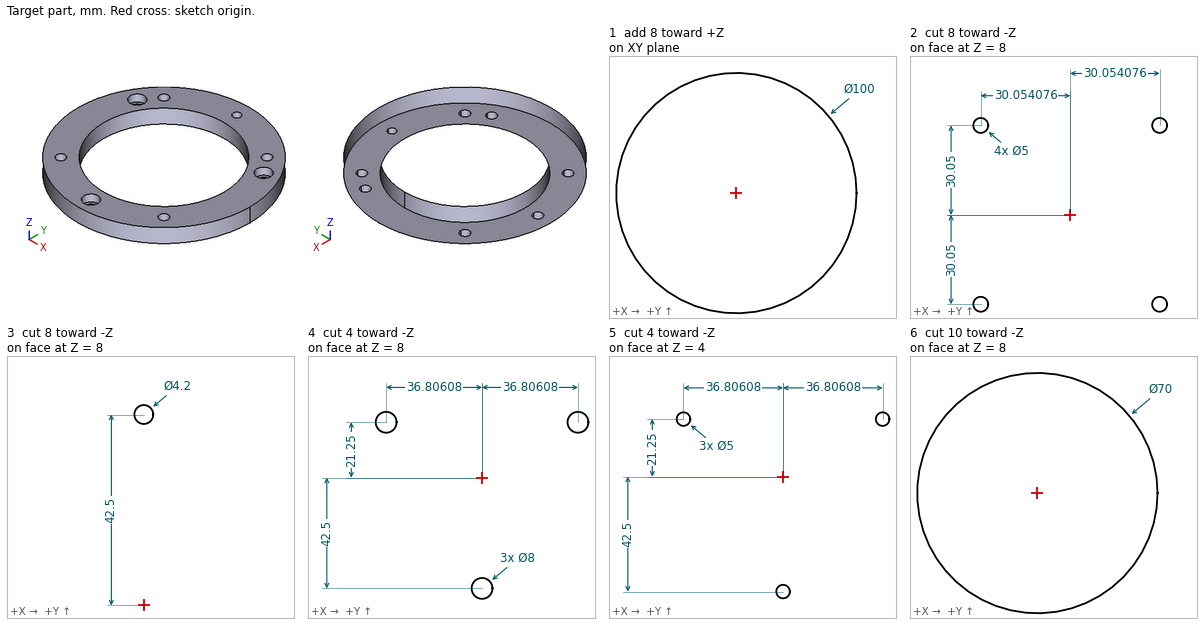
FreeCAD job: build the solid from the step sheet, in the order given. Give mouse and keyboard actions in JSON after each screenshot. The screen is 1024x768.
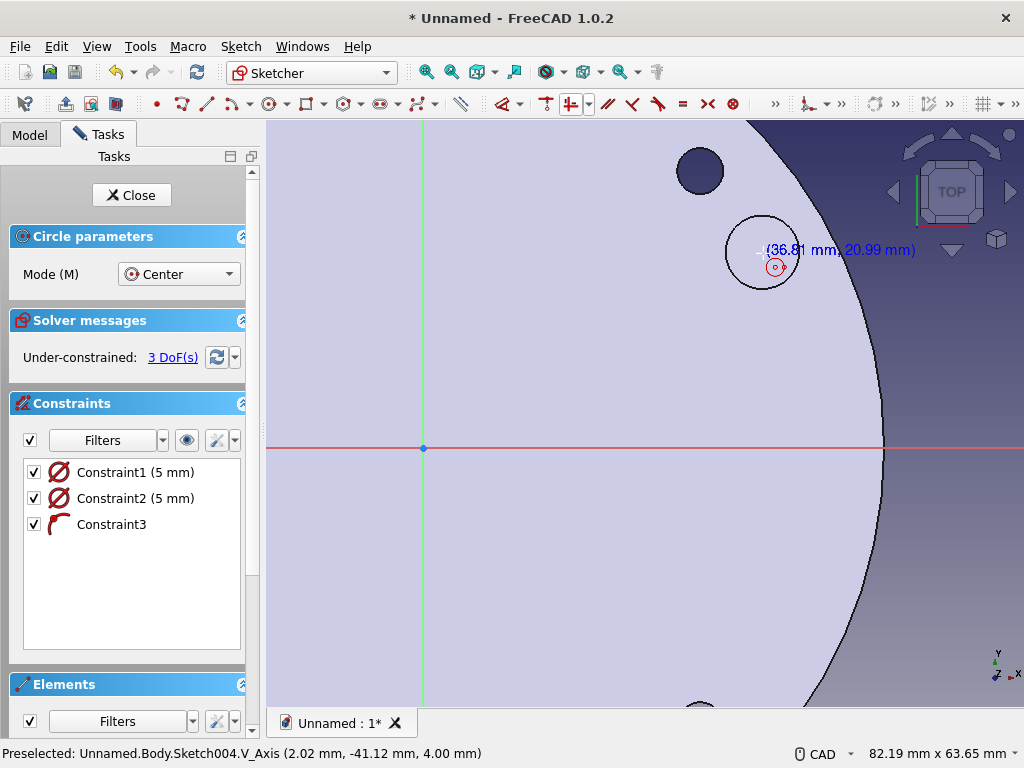
{"action": "left_click", "coordinate": [762, 252]}
{"action": "mouse_move", "coordinate": [779, 236]}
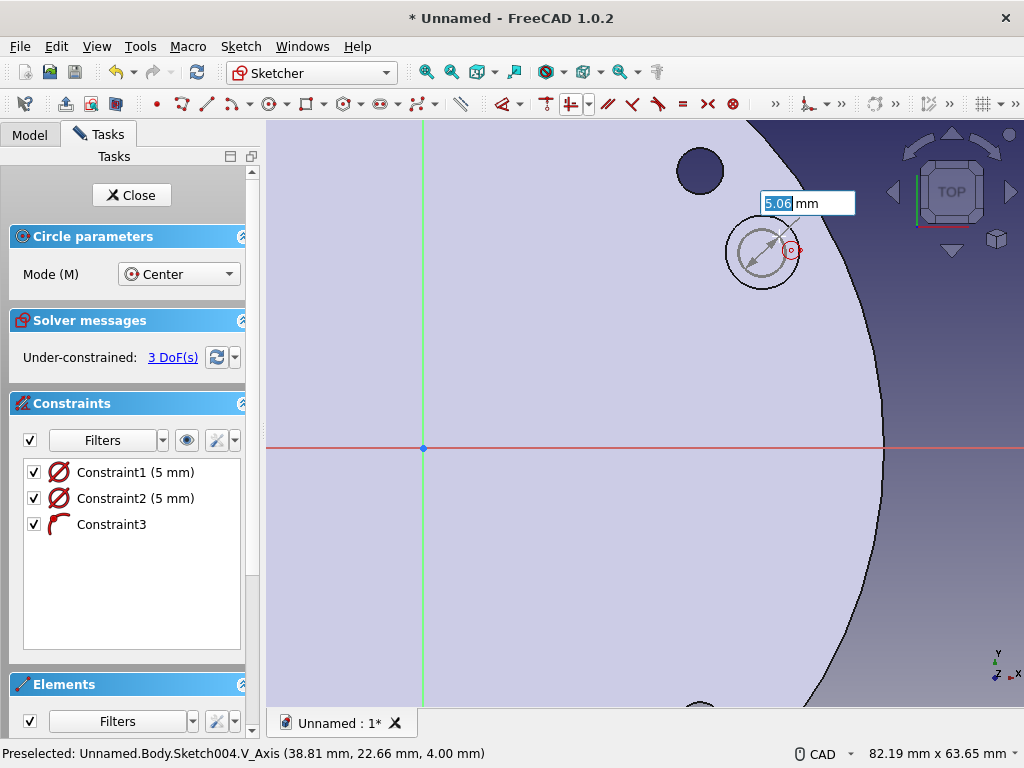
{"action": "type", "text": "5"}
{"action": "key", "text": "Return"}
{"action": "key", "text": "Escape"}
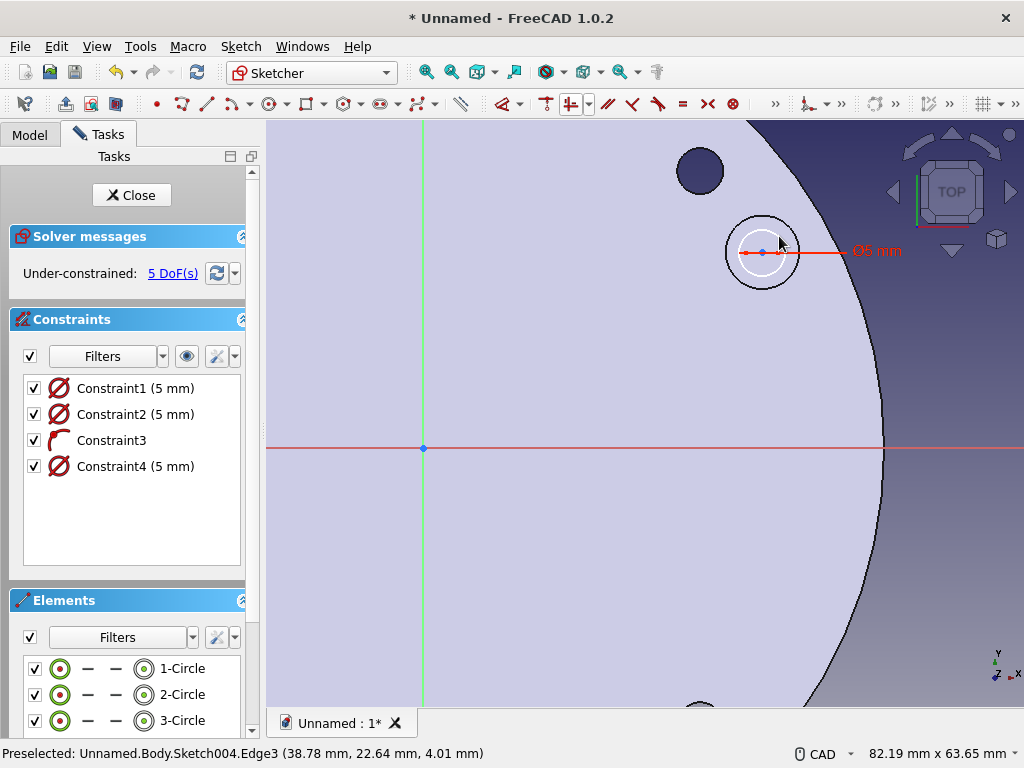
{"action": "scroll", "coordinate": [763, 252], "scroll_direction": "down", "scroll_amount": 3}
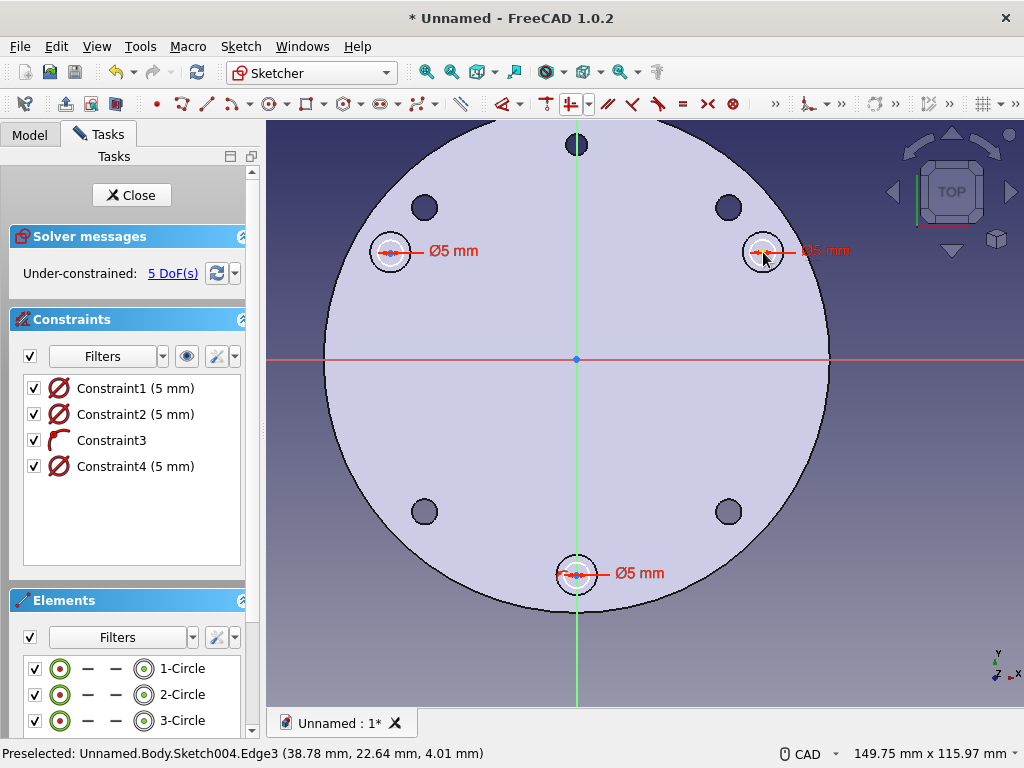
{"action": "left_click", "coordinate": [391, 253]}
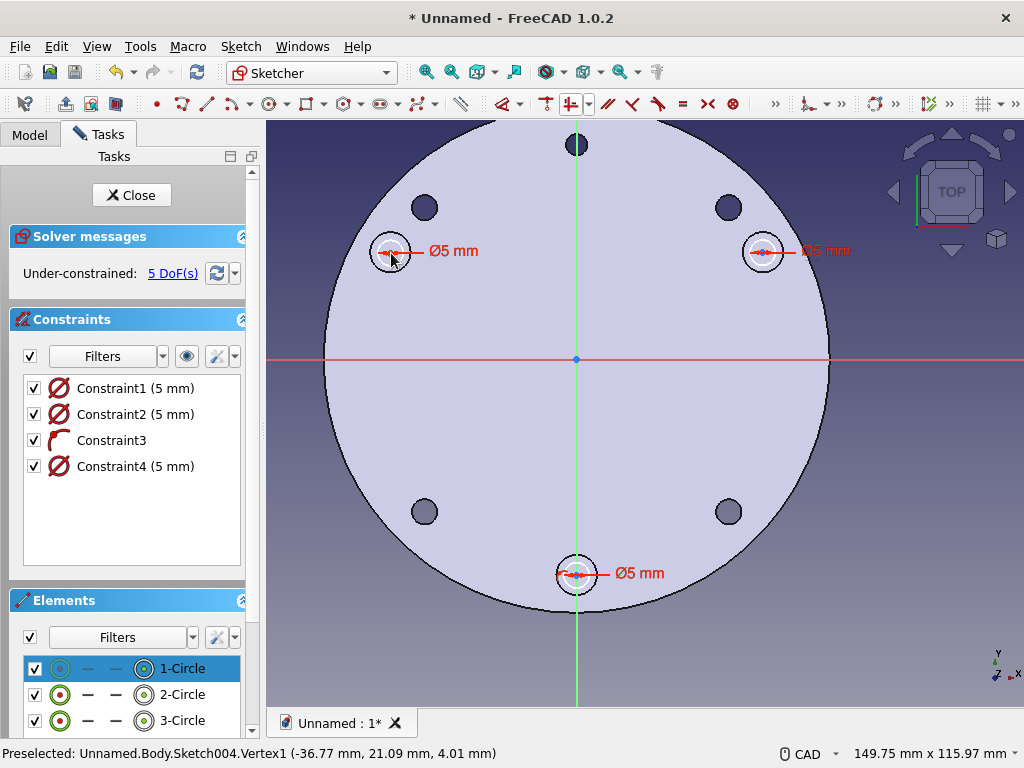
{"action": "left_click", "coordinate": [763, 253]}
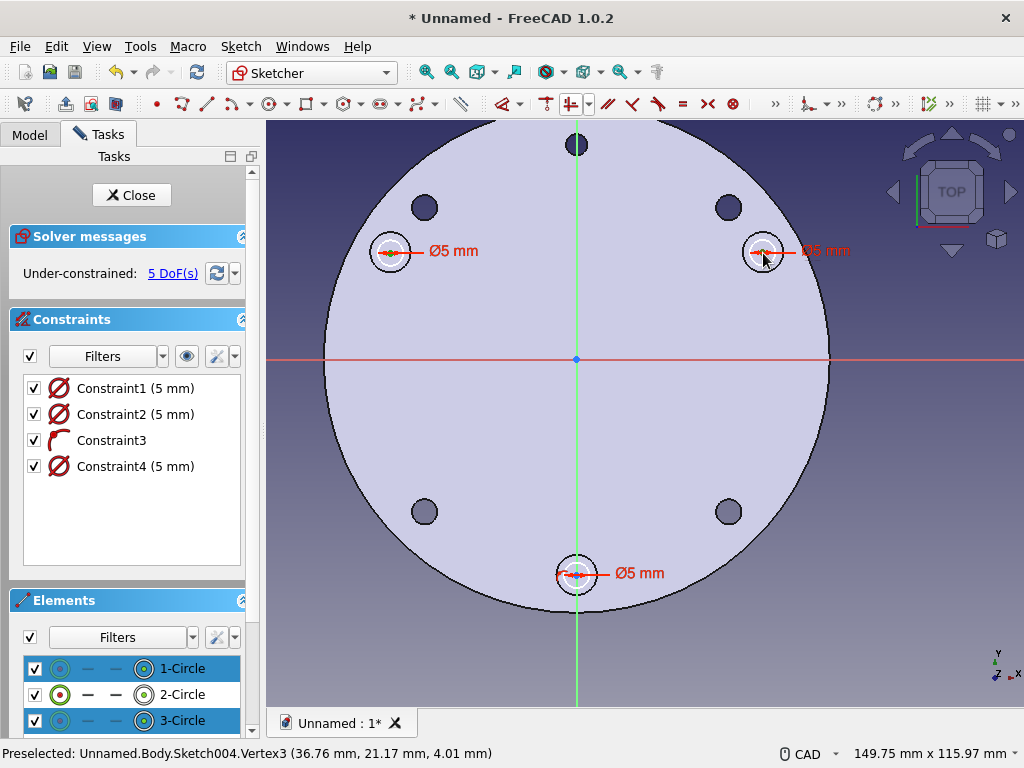
{"action": "left_click", "coordinate": [588, 104]}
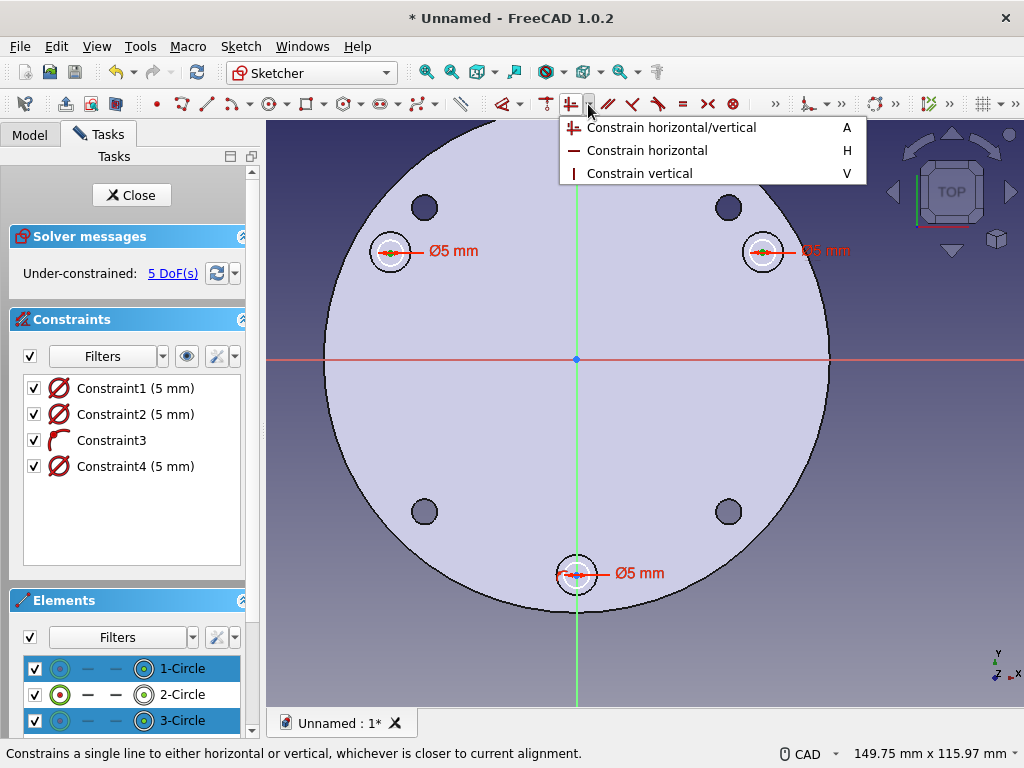
{"action": "left_click", "coordinate": [713, 150]}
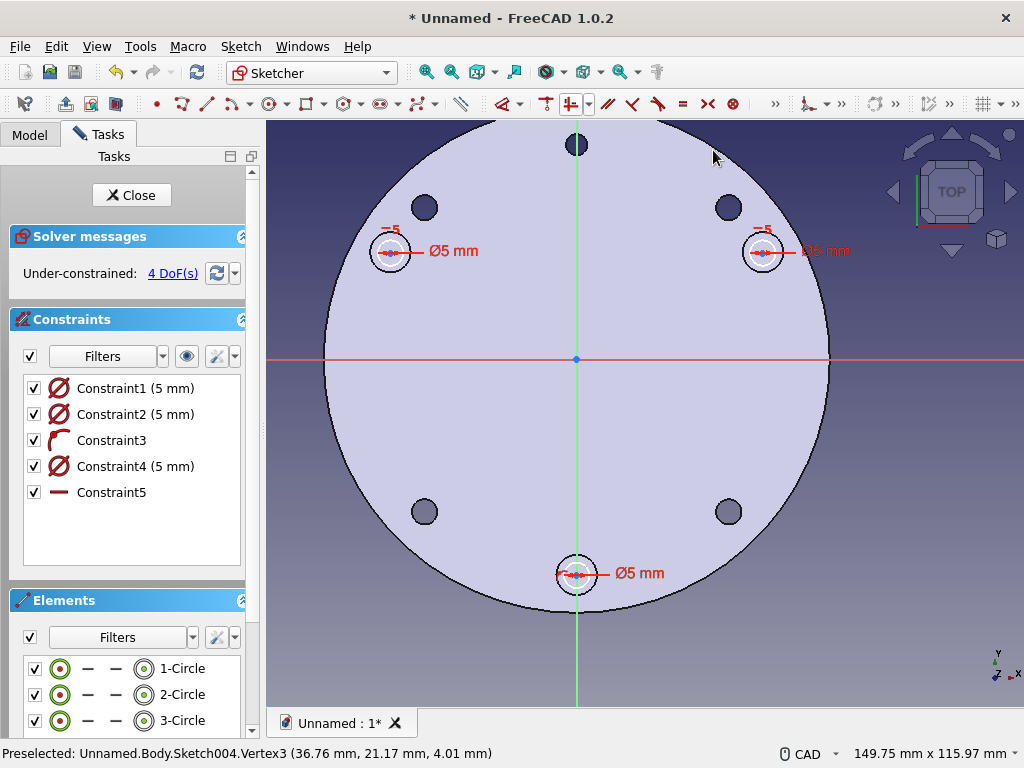
{"action": "left_click", "coordinate": [502, 104]}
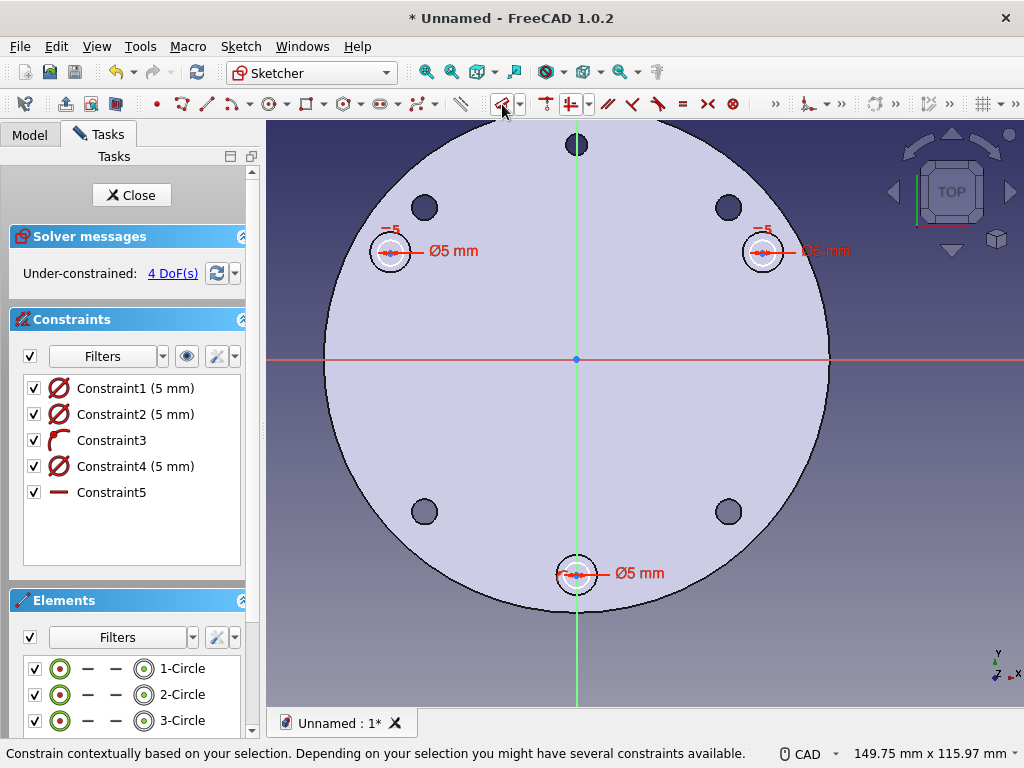
{"action": "left_click", "coordinate": [577, 575]}
{"action": "left_click", "coordinate": [611, 468]}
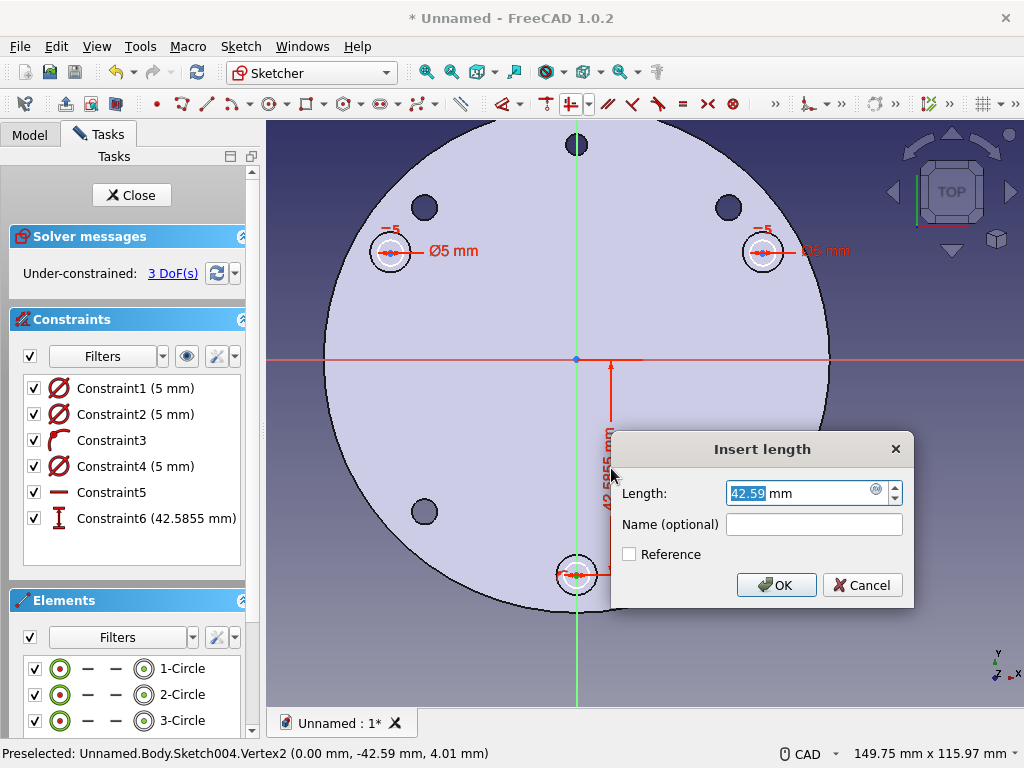
{"action": "type", "text": "42.5"}
{"action": "key", "text": "Return"}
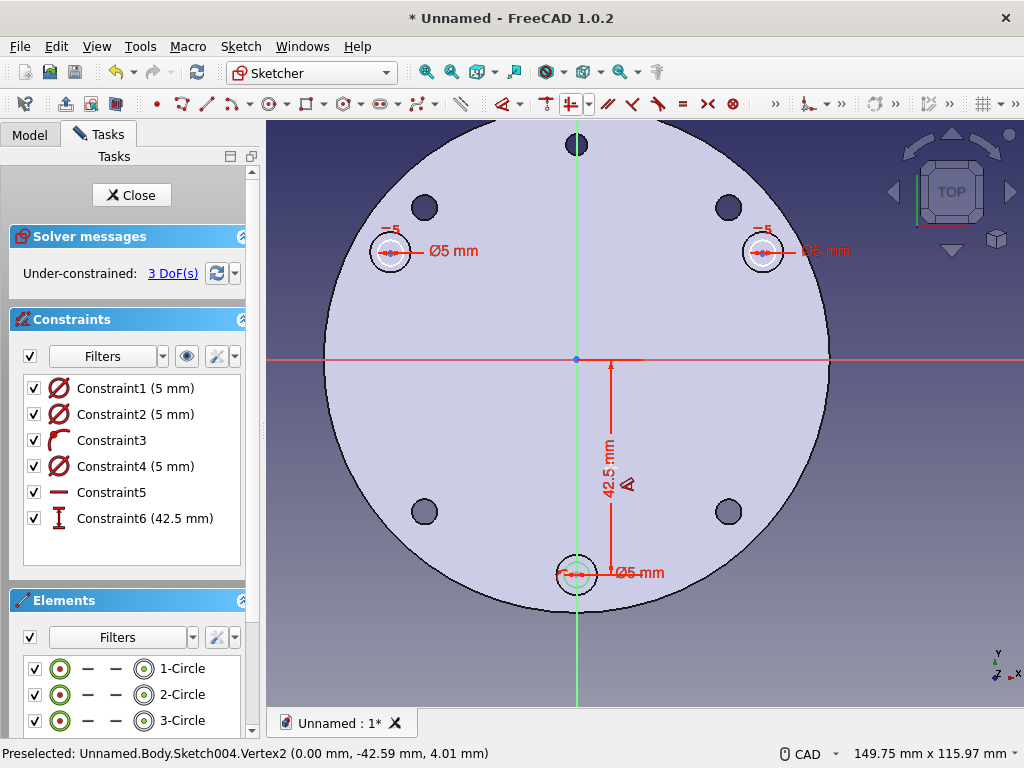
{"action": "left_click", "coordinate": [391, 253]}
{"action": "left_click", "coordinate": [357, 306]}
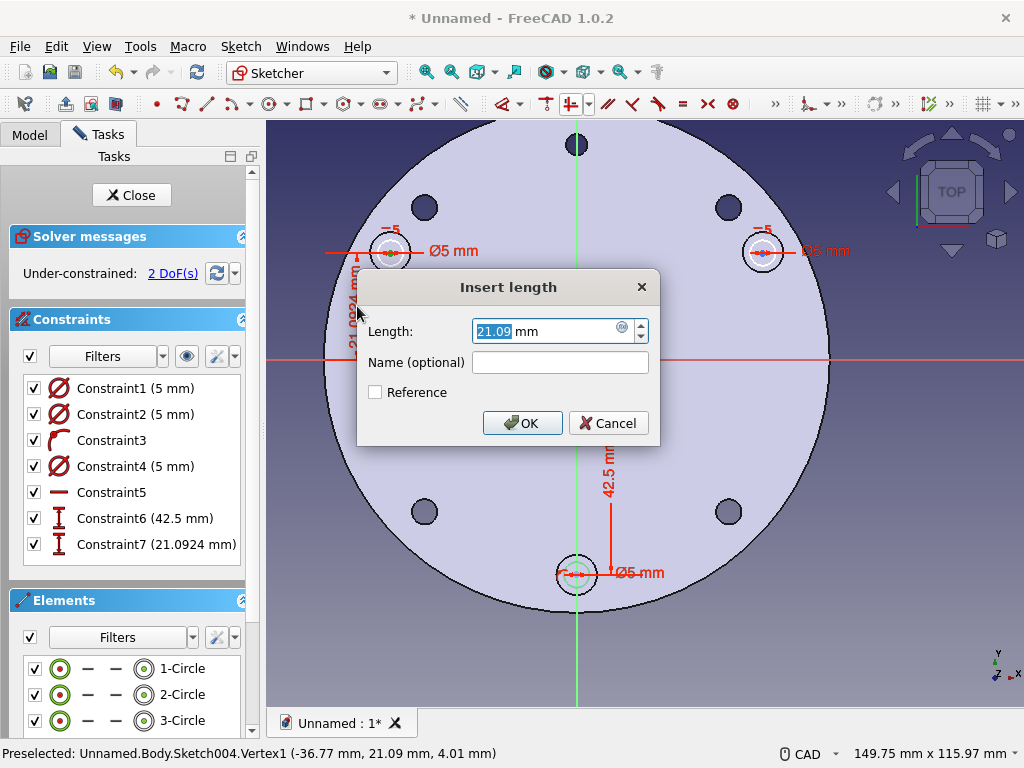
{"action": "type", "text": "21.25"}
{"action": "key", "text": "Return"}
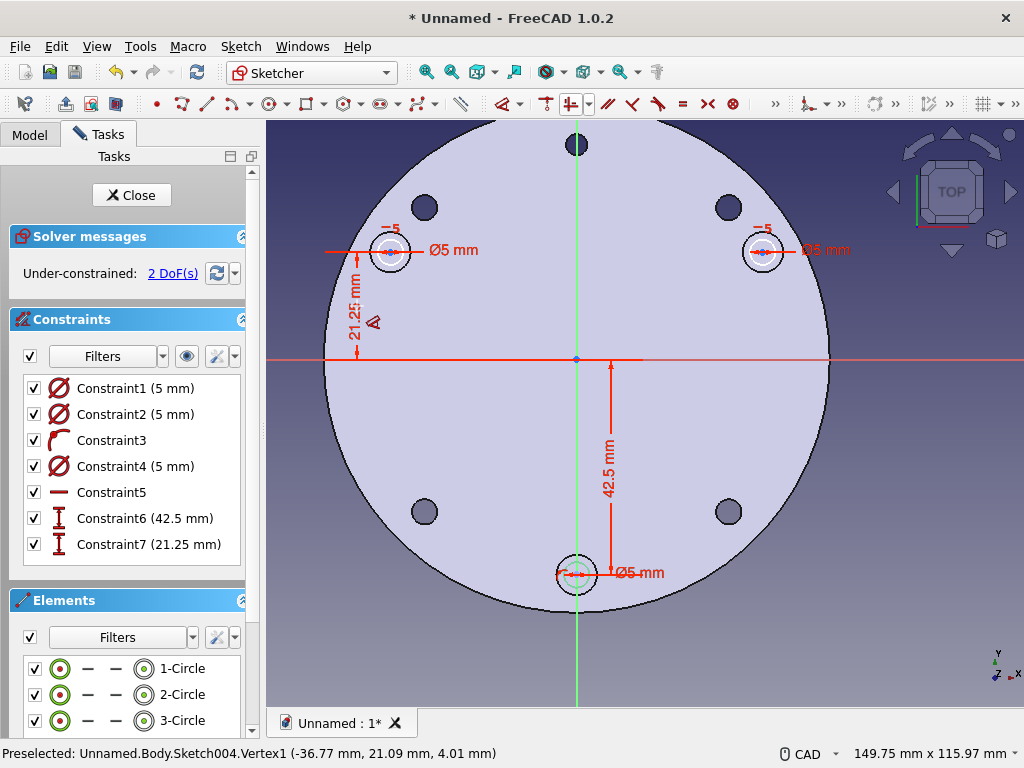
{"action": "left_click", "coordinate": [391, 252]}
{"action": "left_click", "coordinate": [484, 218]}